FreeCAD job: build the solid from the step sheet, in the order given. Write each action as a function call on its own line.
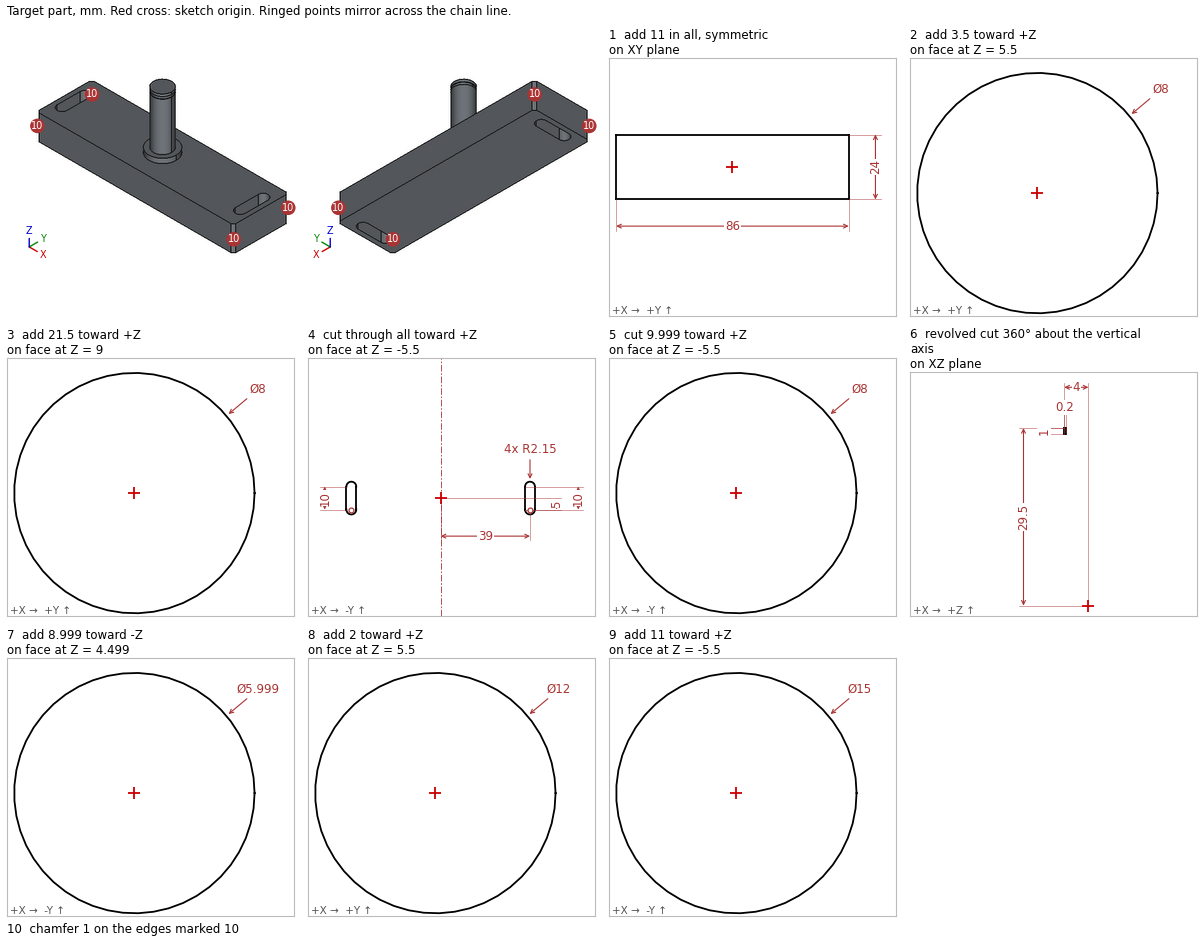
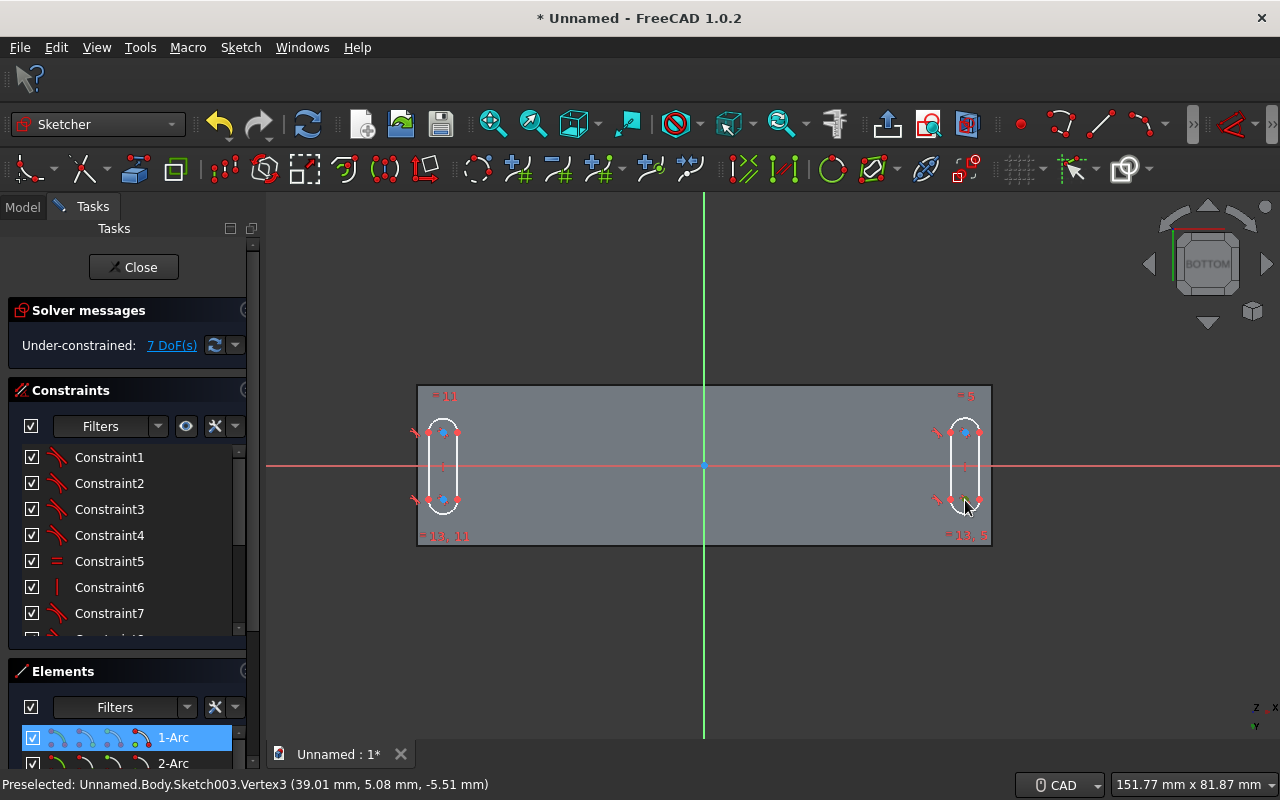
click(443, 500)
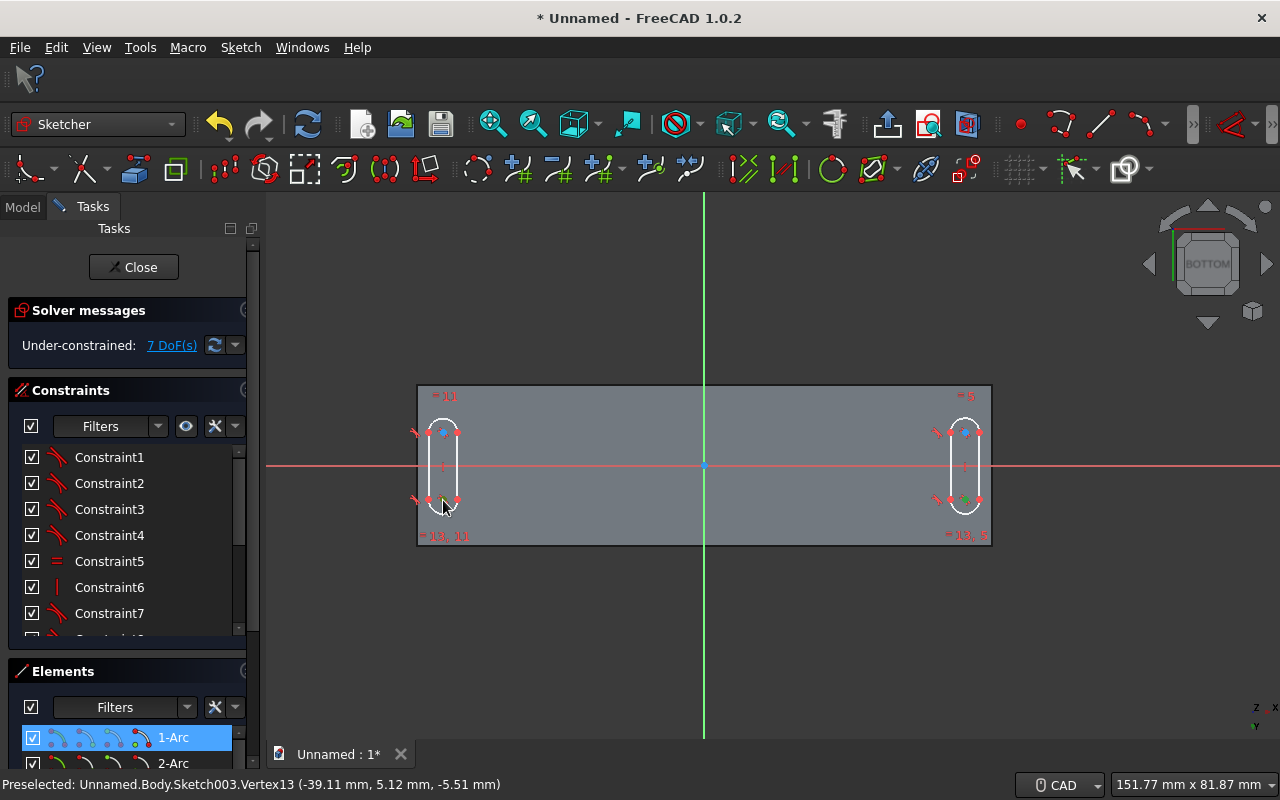
click(704, 676)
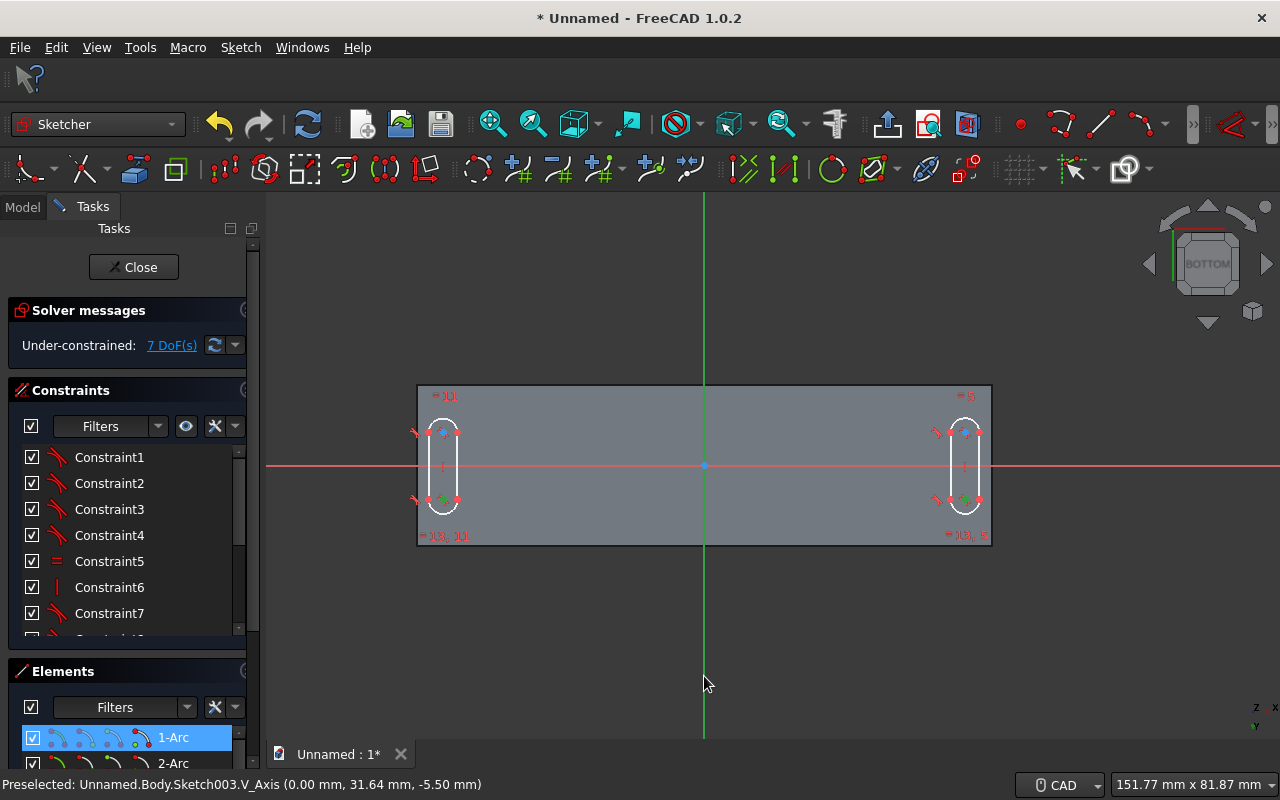
key(s)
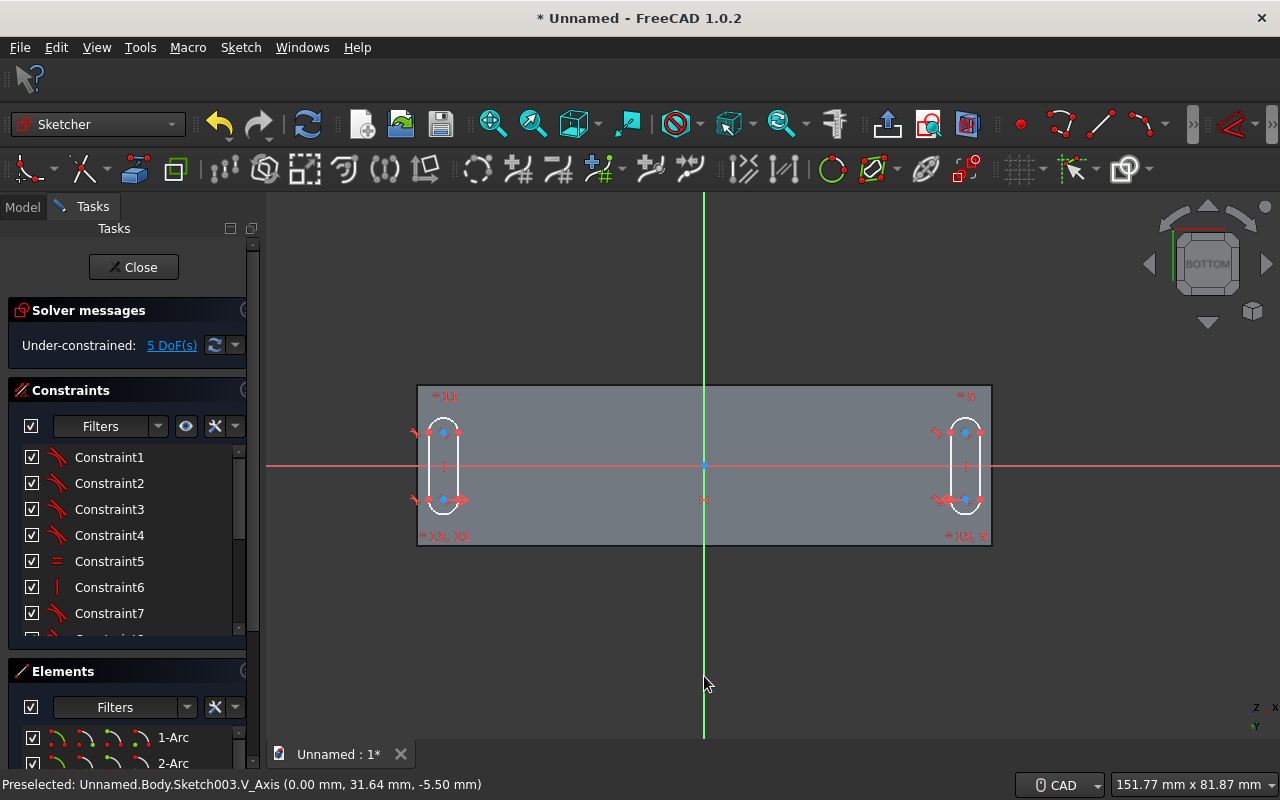
scroll(957, 512, up, 6)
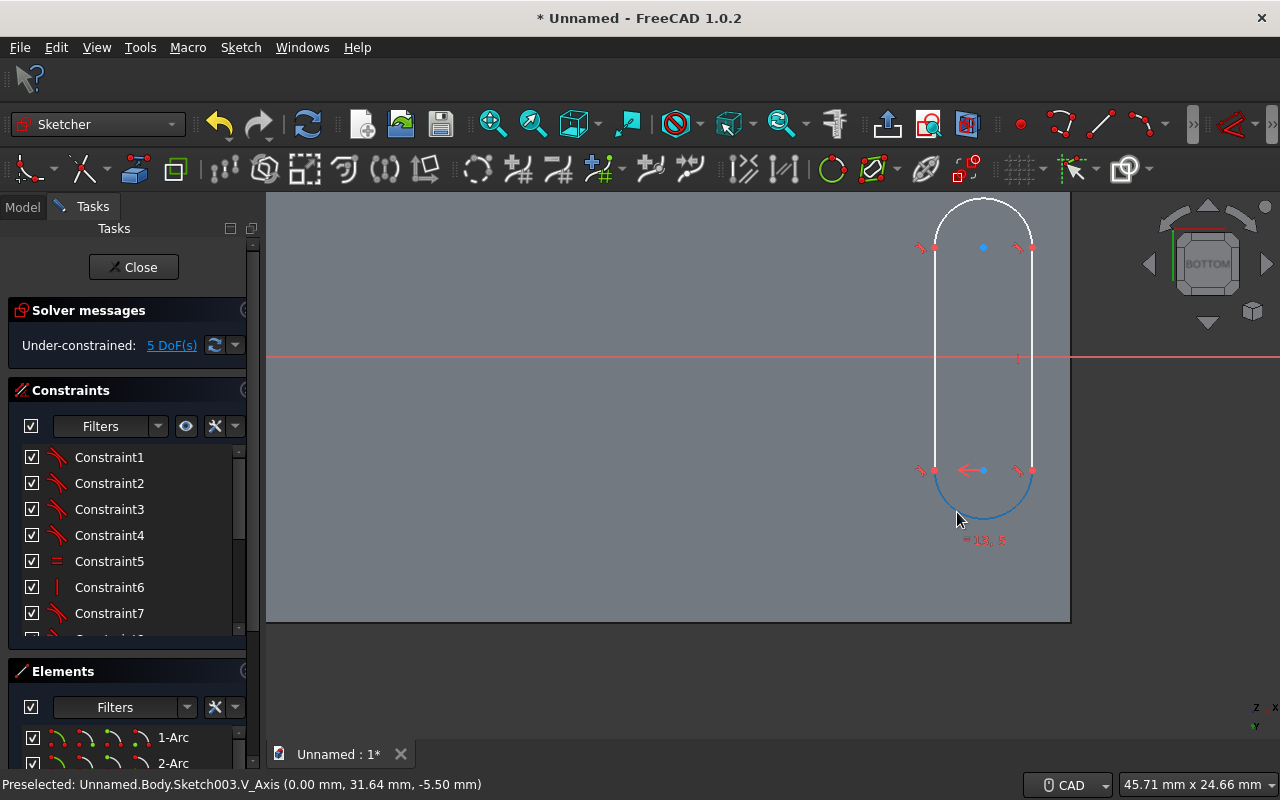
click(955, 510)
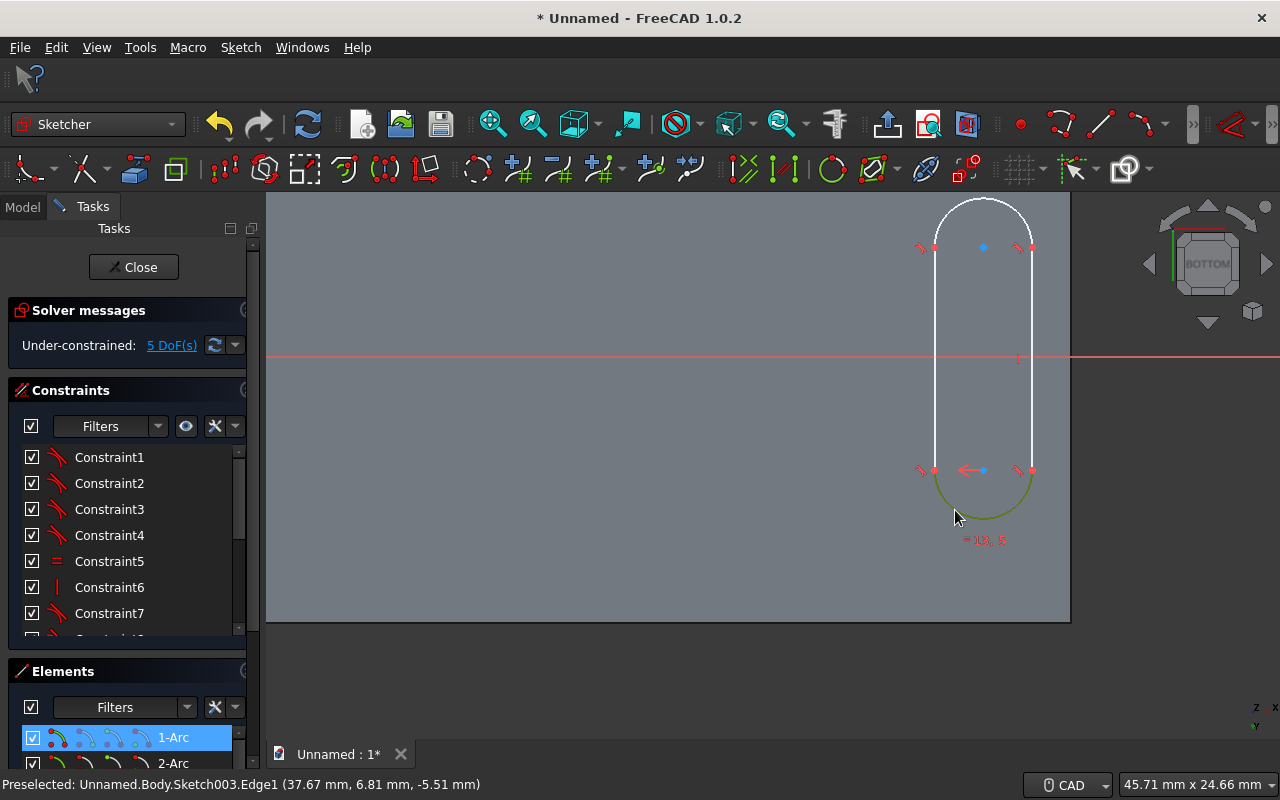
click(1258, 124)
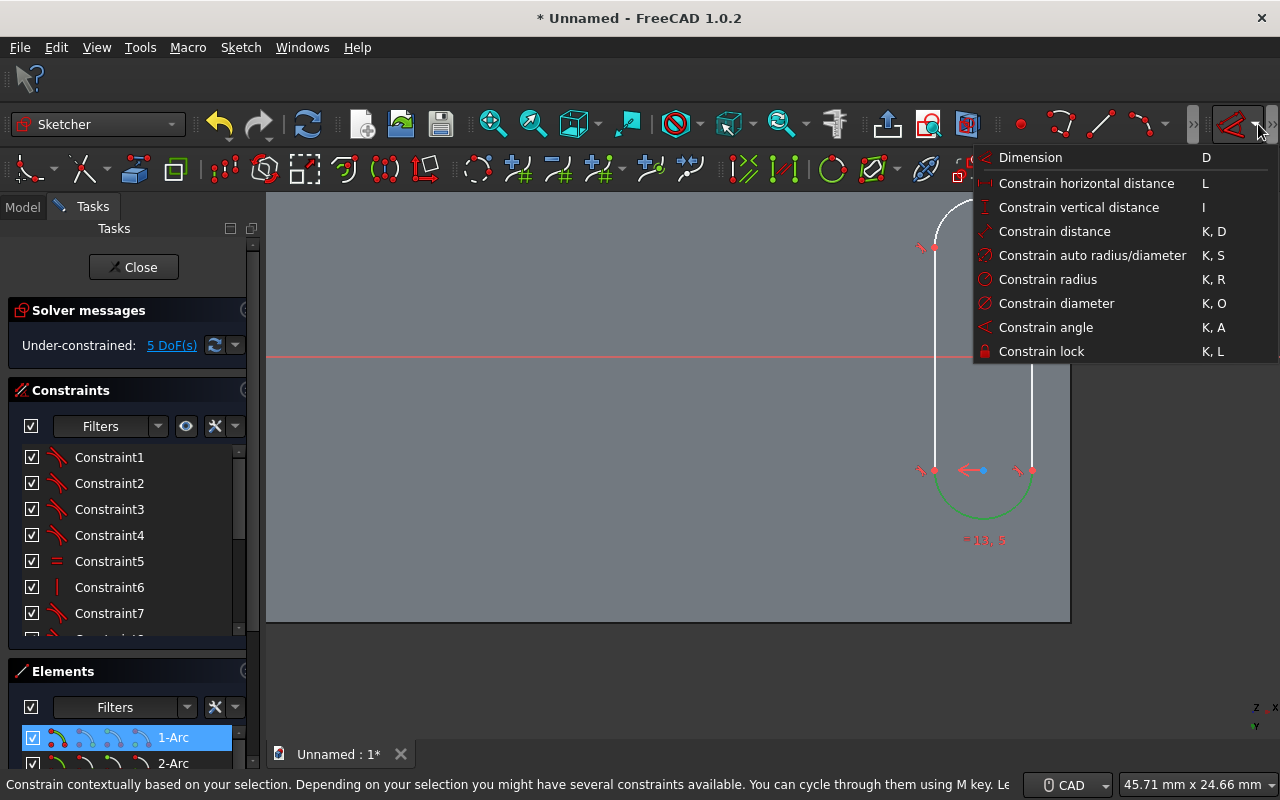
click(1126, 279)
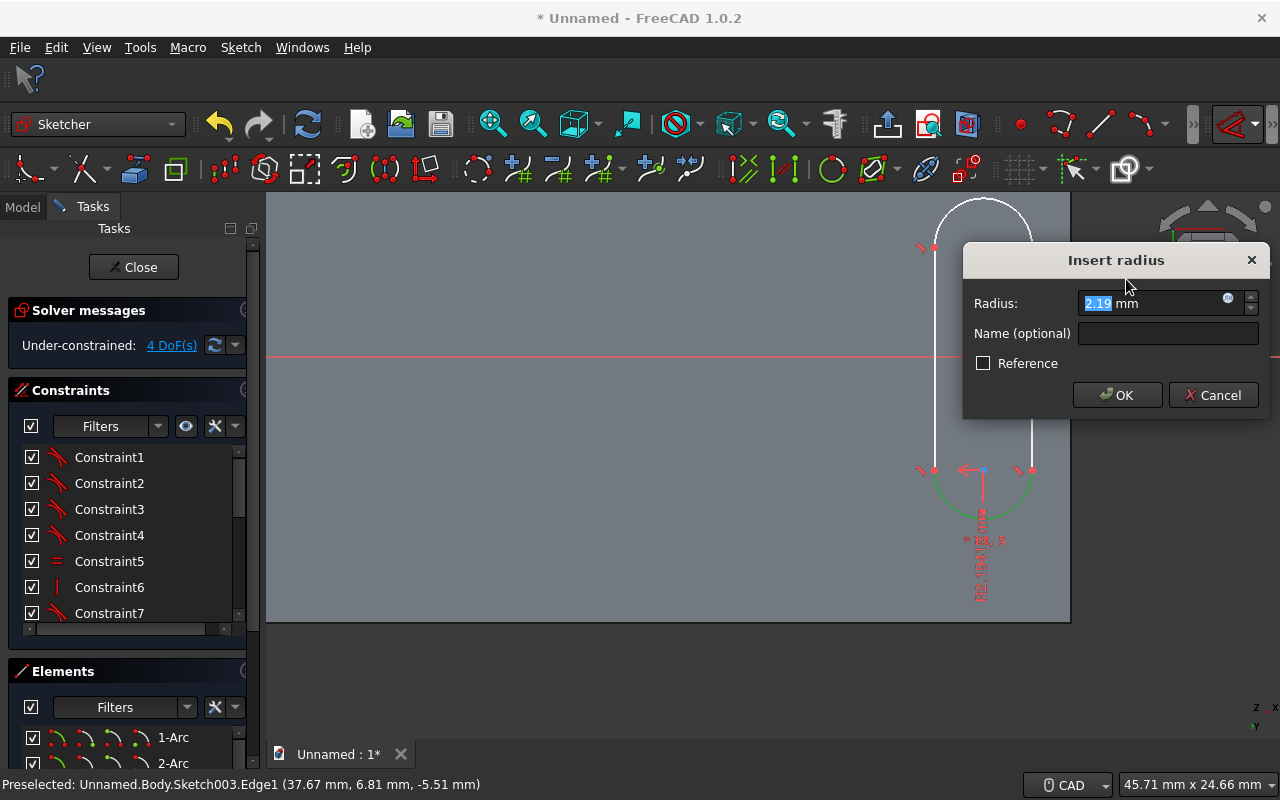
text(2.15)
key(Return)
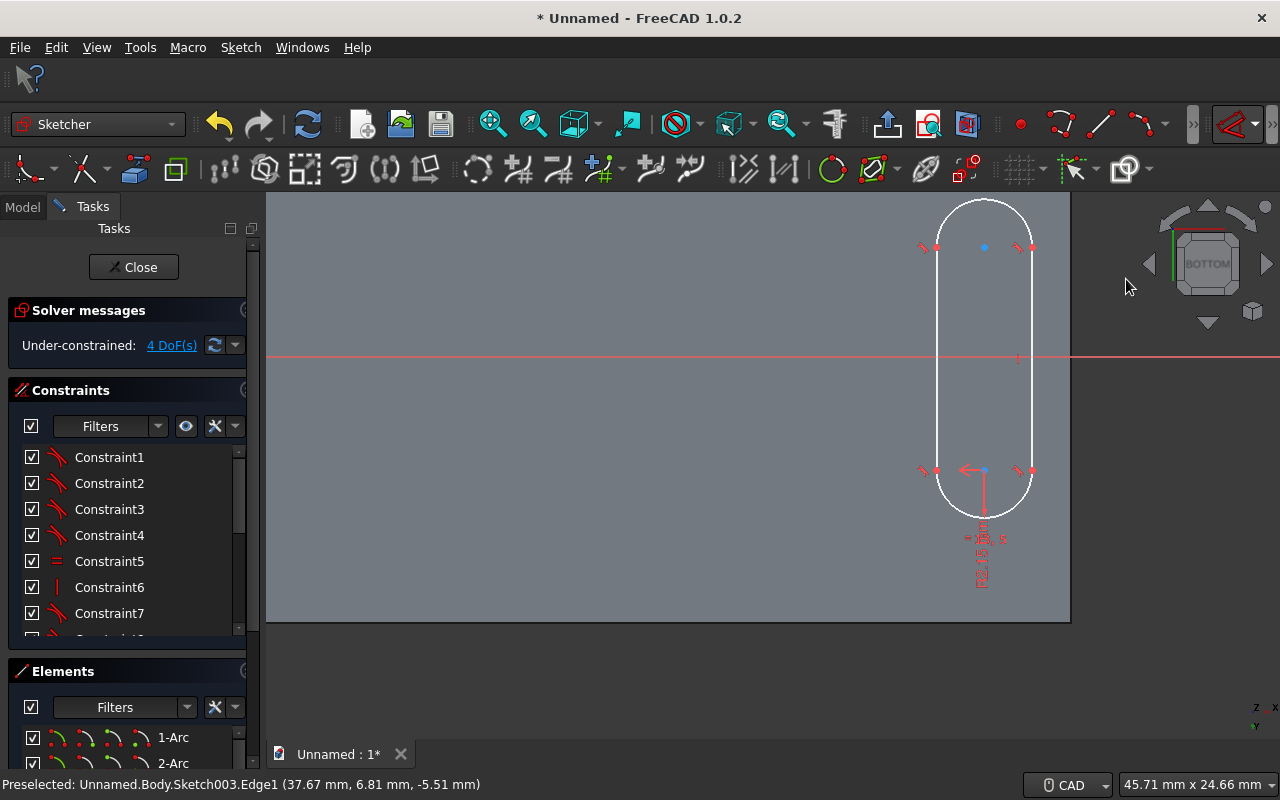
scroll(958, 512, down, 6)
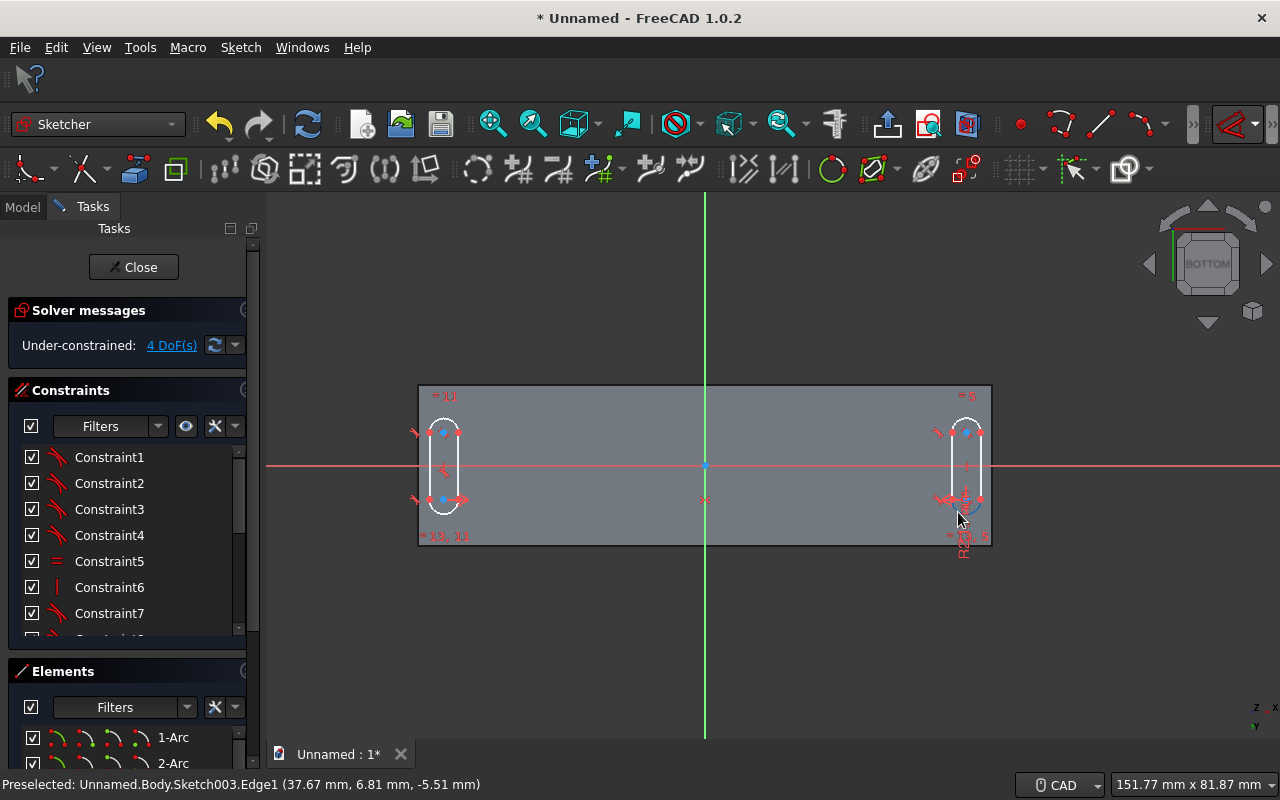
click(952, 480)